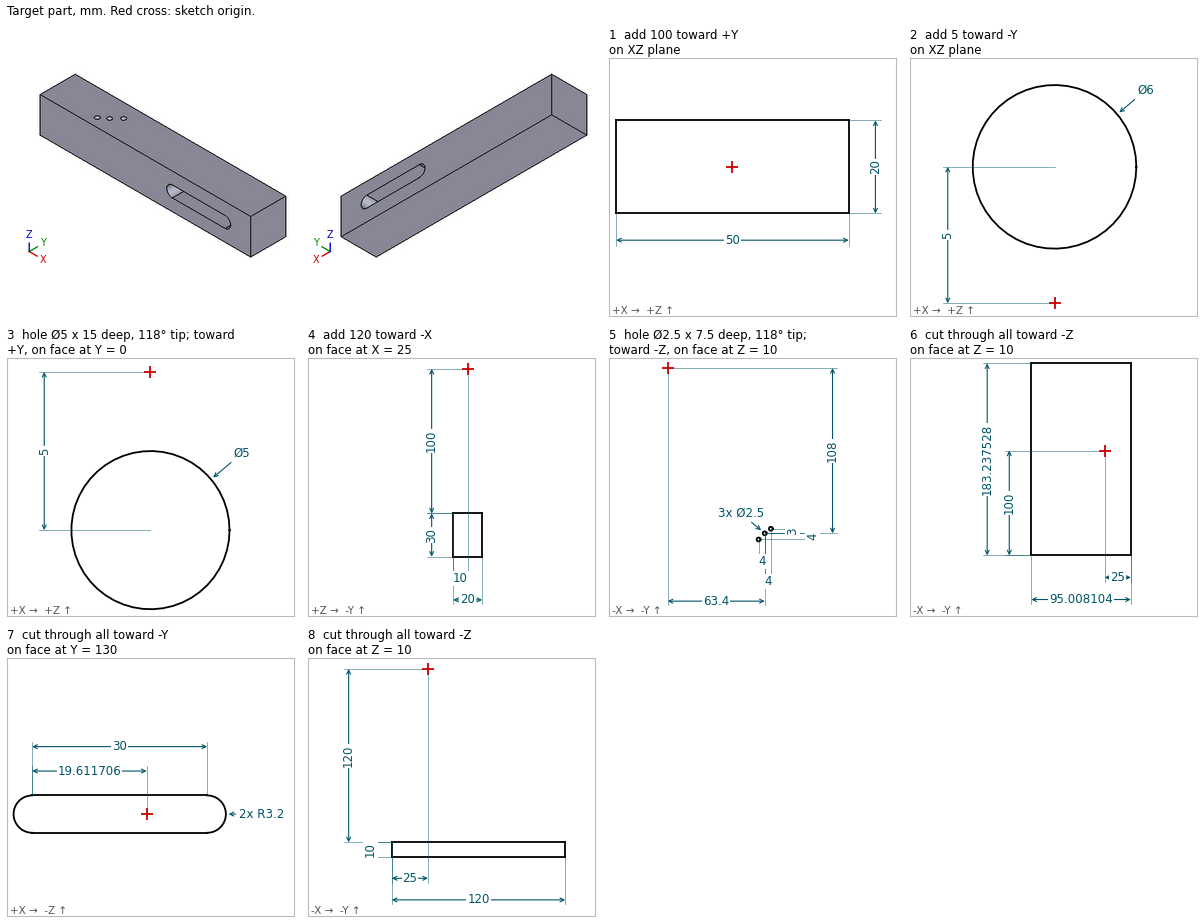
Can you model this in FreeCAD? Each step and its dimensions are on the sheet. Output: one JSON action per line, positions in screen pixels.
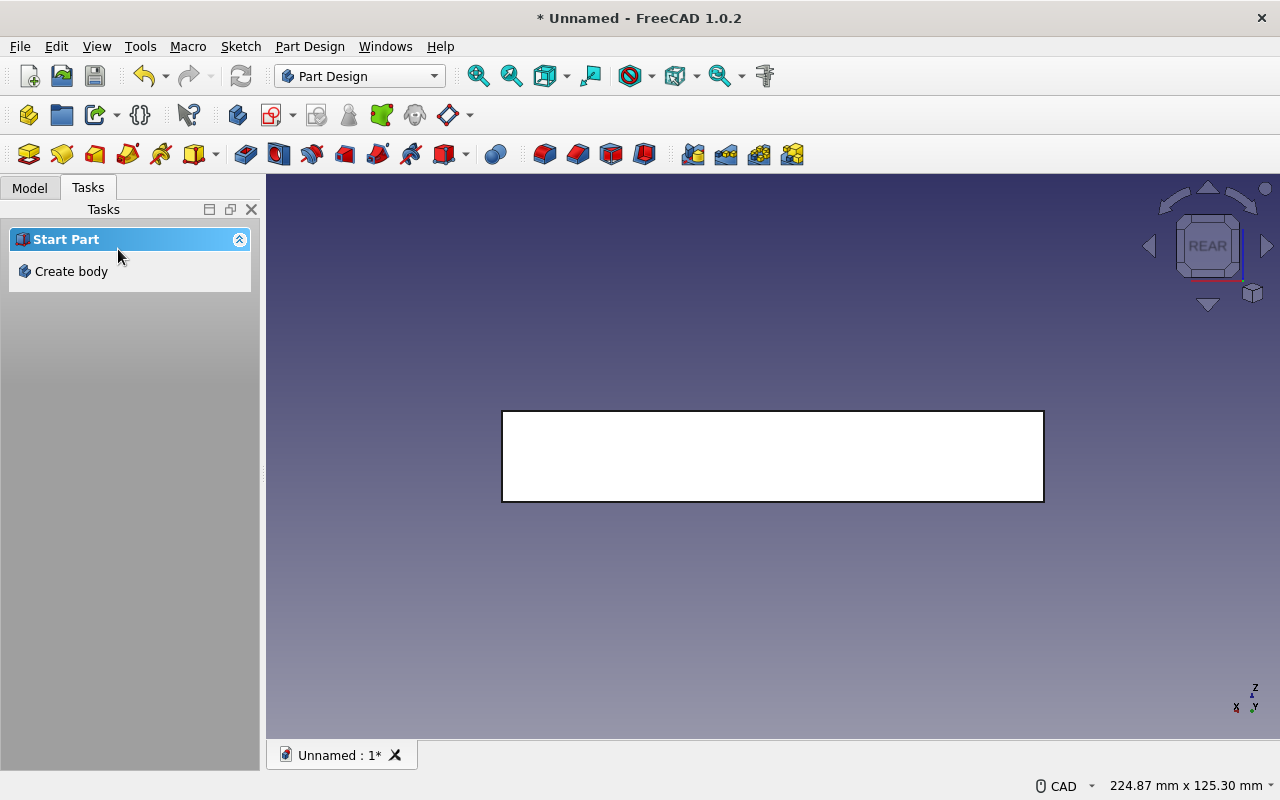
{"action": "left_click", "coordinate": [618, 456]}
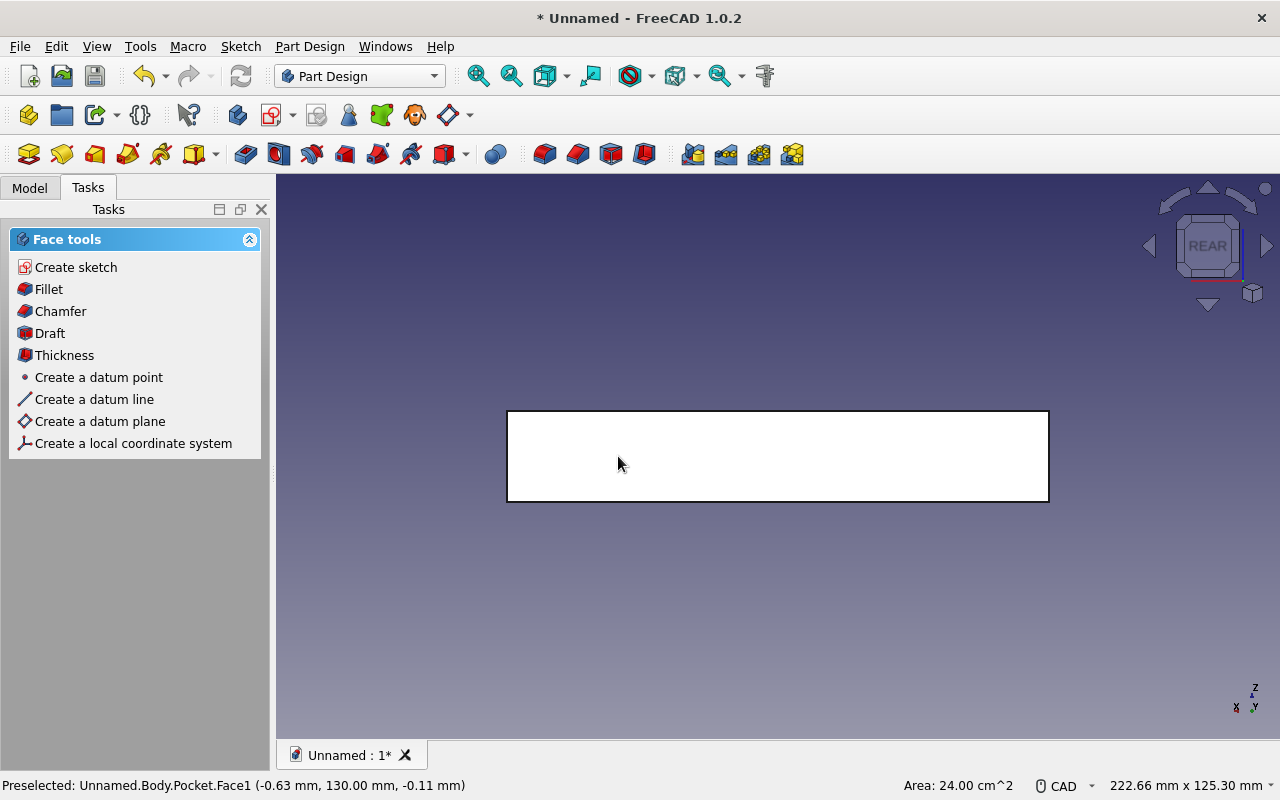
{"action": "left_click", "coordinate": [270, 116]}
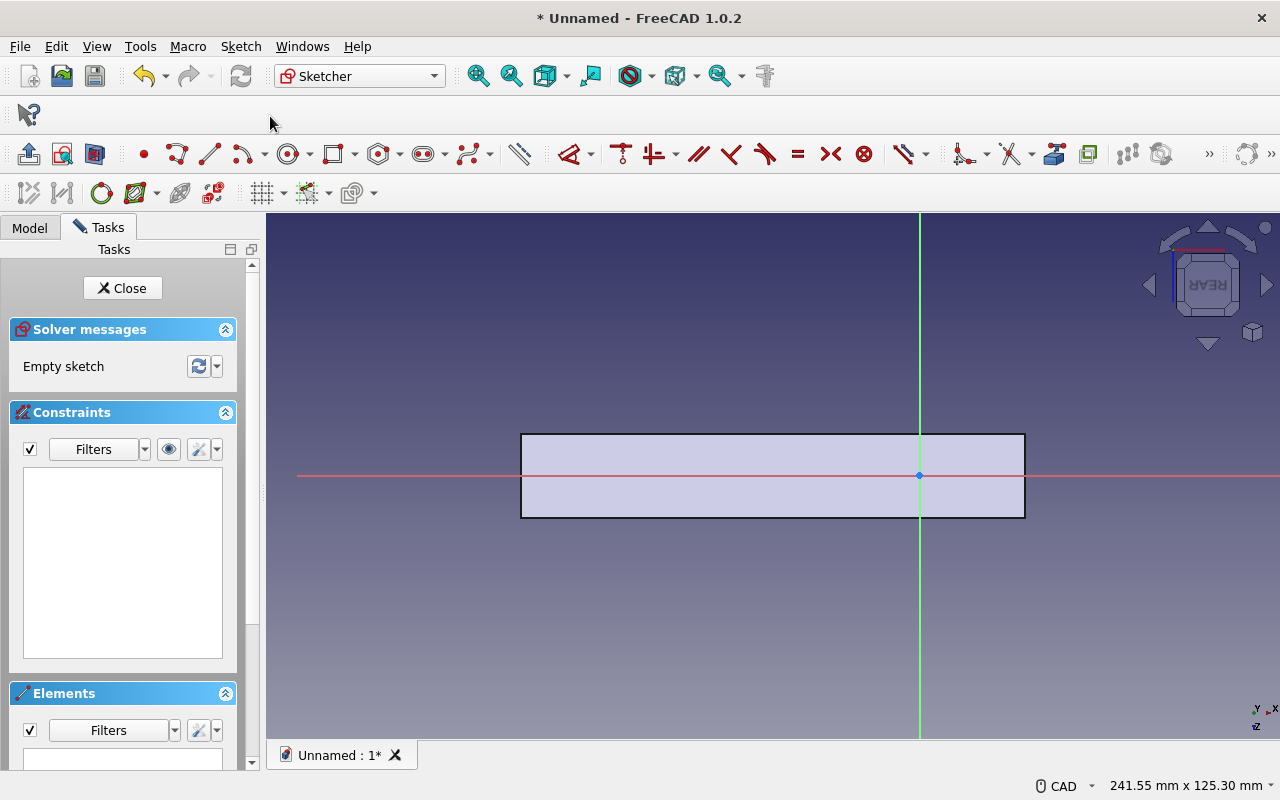
{"action": "scroll", "coordinate": [965, 476], "scroll_direction": "up", "scroll_amount": 7}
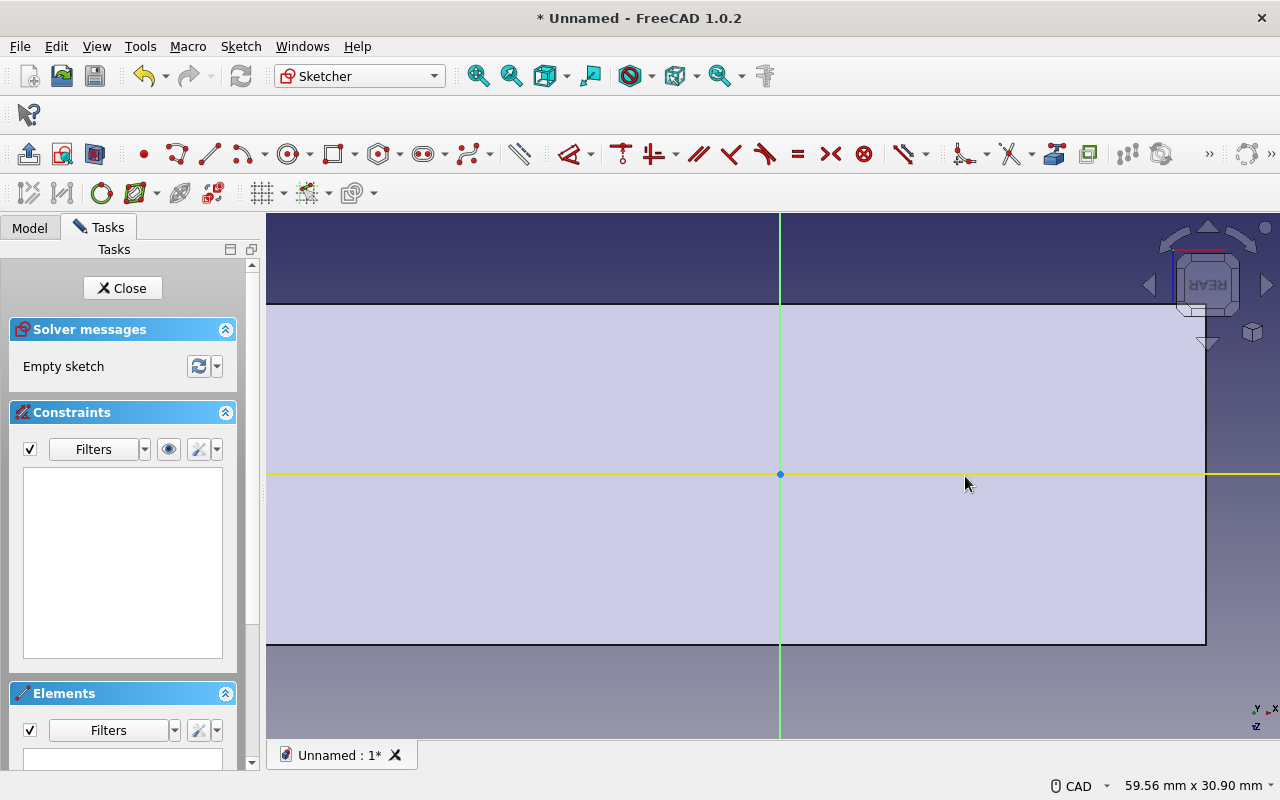
{"action": "key", "text": "g s"}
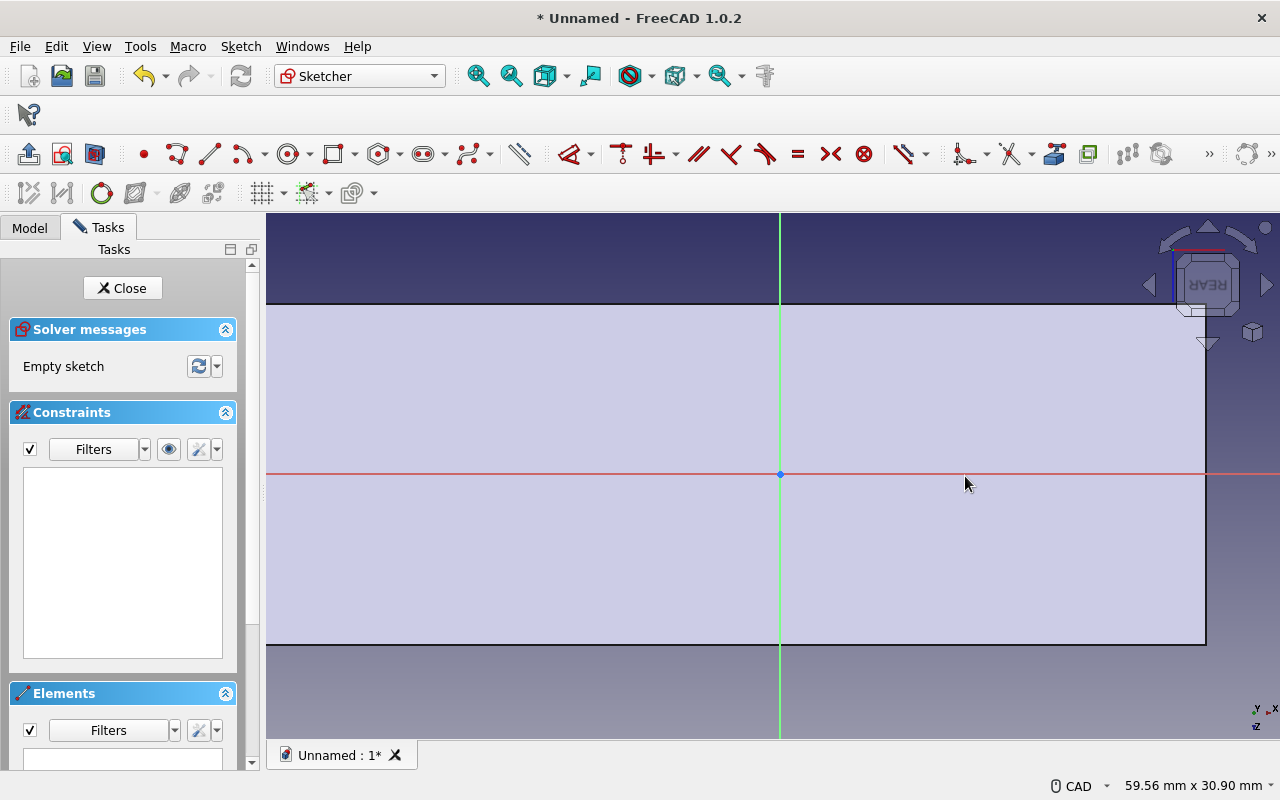
{"action": "left_click", "coordinate": [446, 474]}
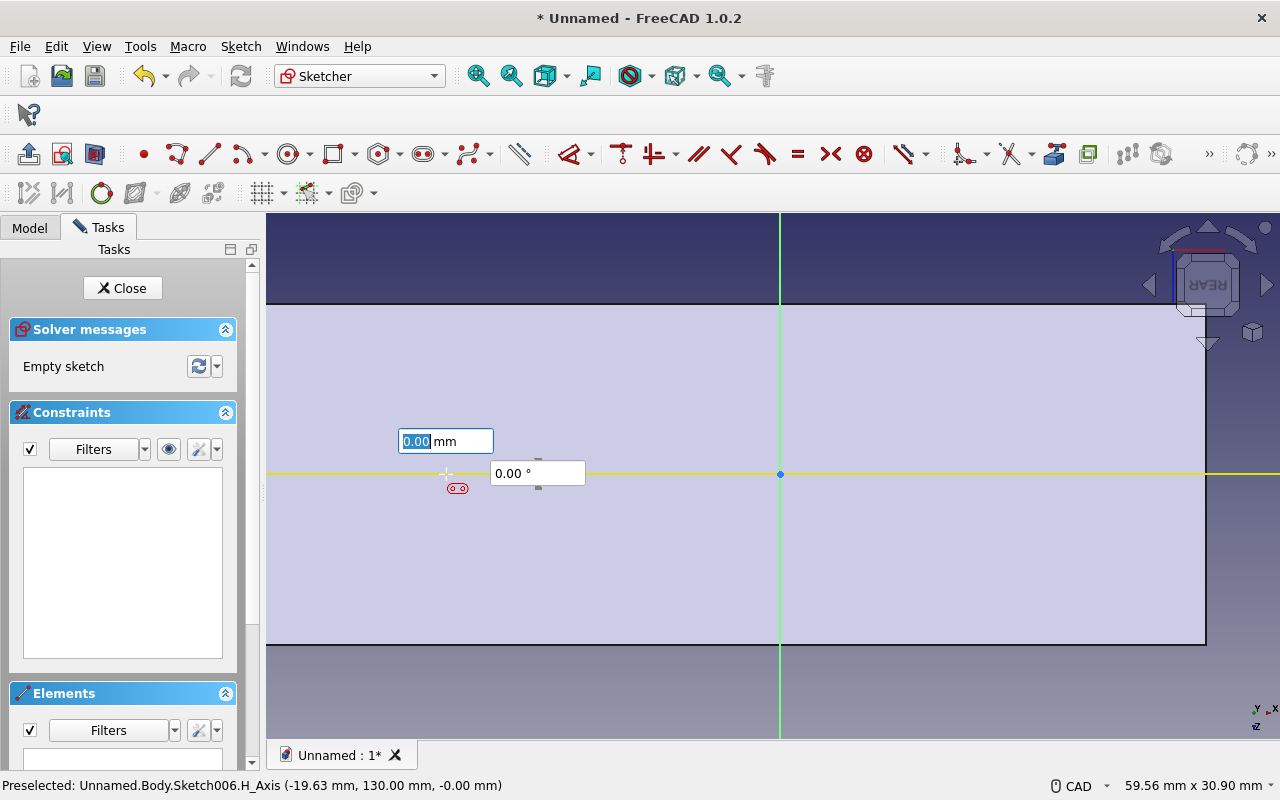
{"action": "left_click", "coordinate": [957, 465]}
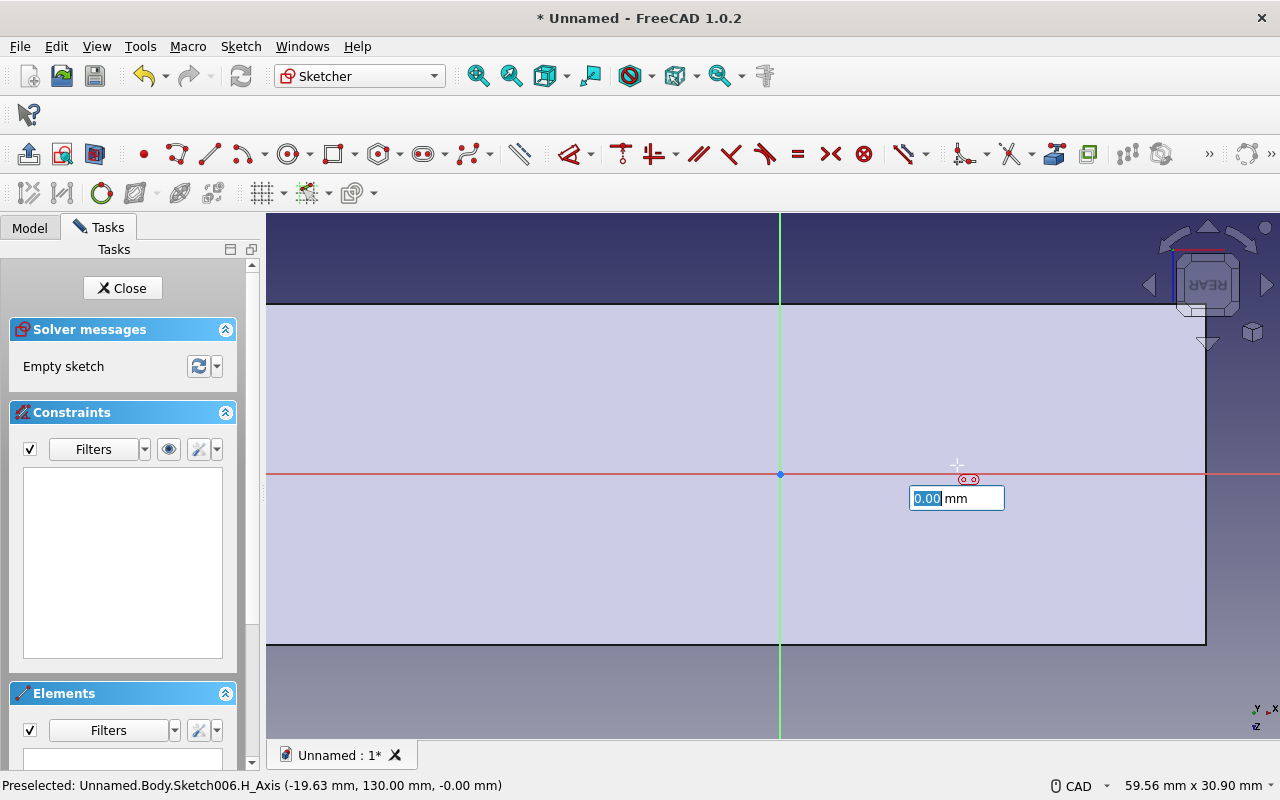
{"action": "left_click", "coordinate": [702, 529]}
{"action": "key", "text": "Escape"}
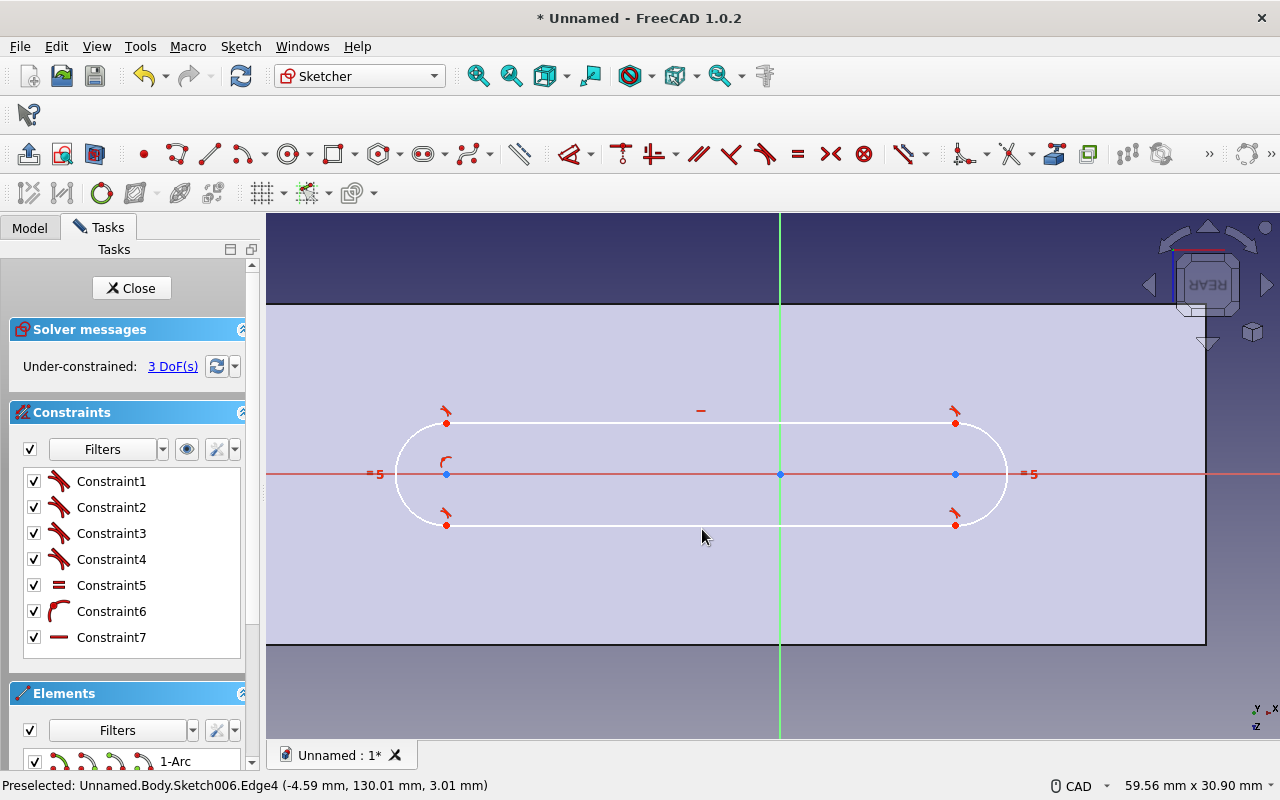
{"action": "left_click", "coordinate": [568, 154]}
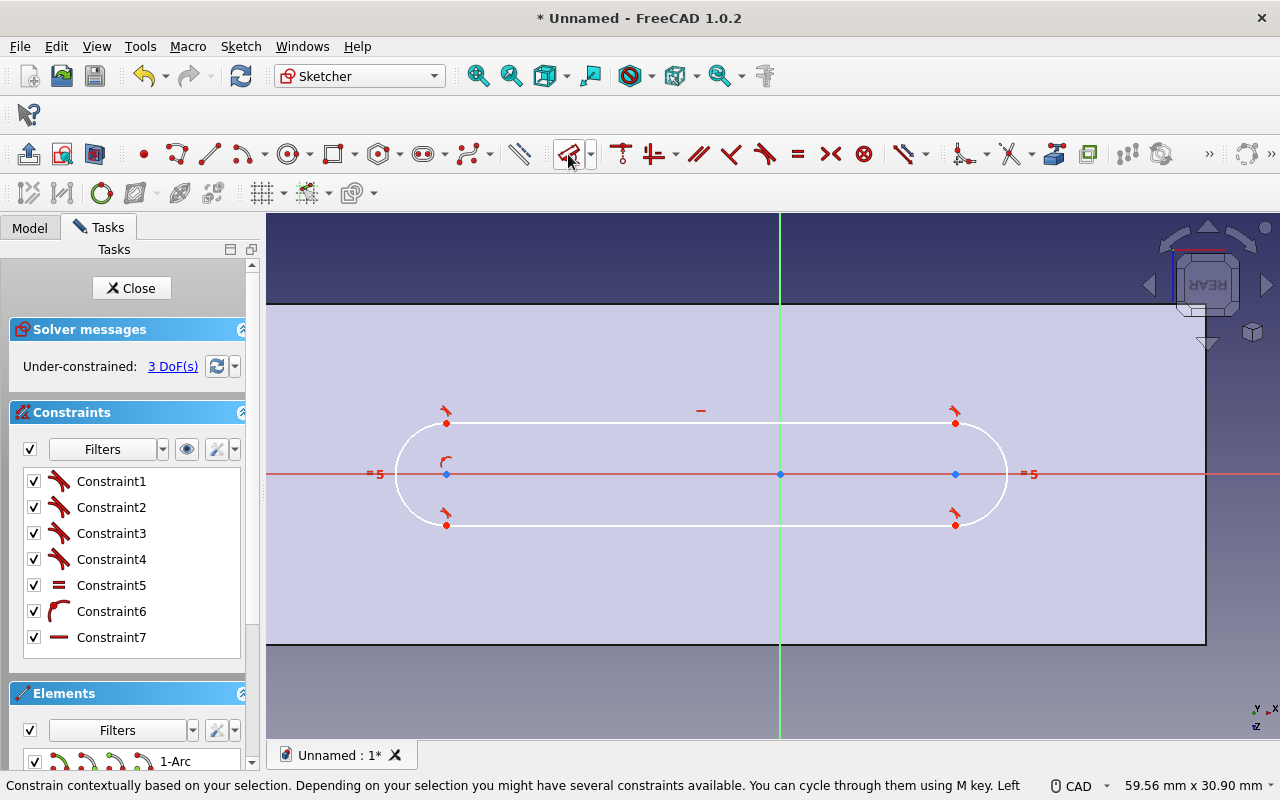
{"action": "left_click", "coordinate": [405, 444]}
{"action": "left_click", "coordinate": [379, 425]}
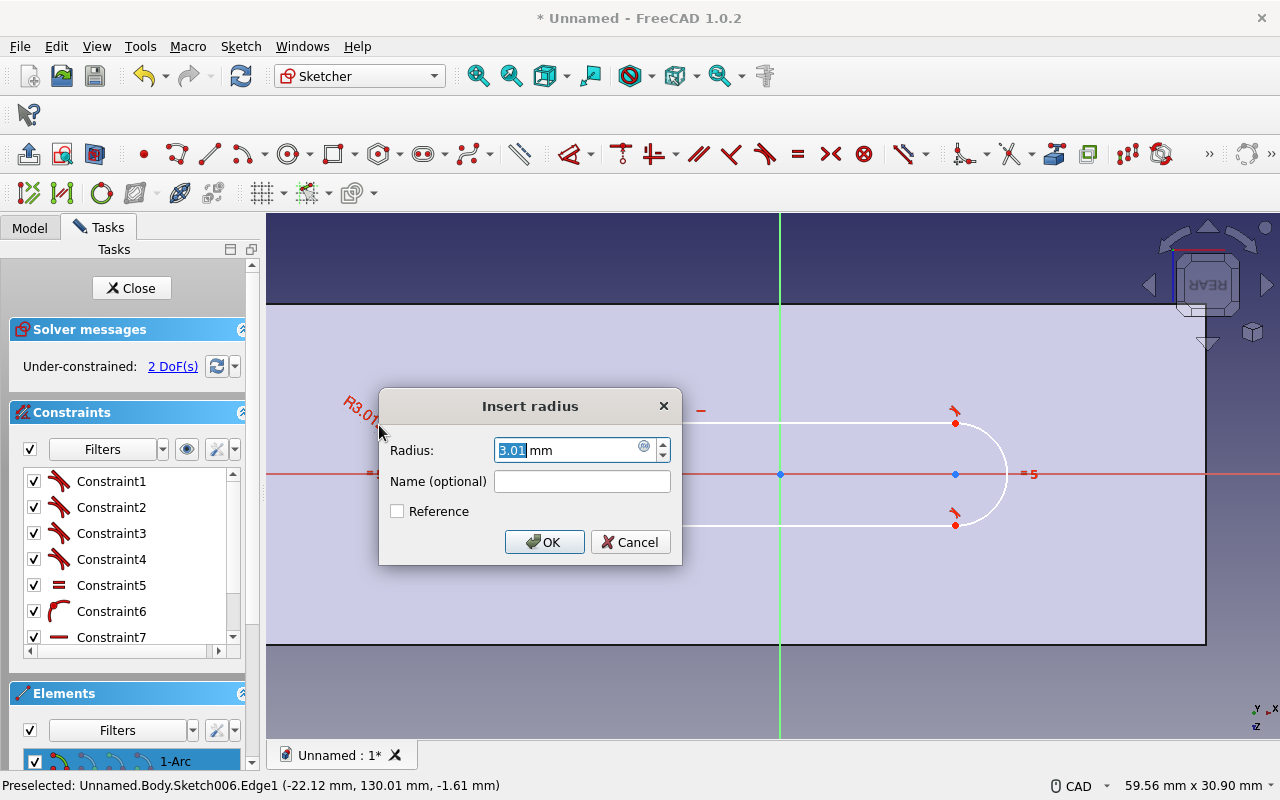
{"action": "type", "text": "3.2"}
{"action": "key", "text": "Return"}